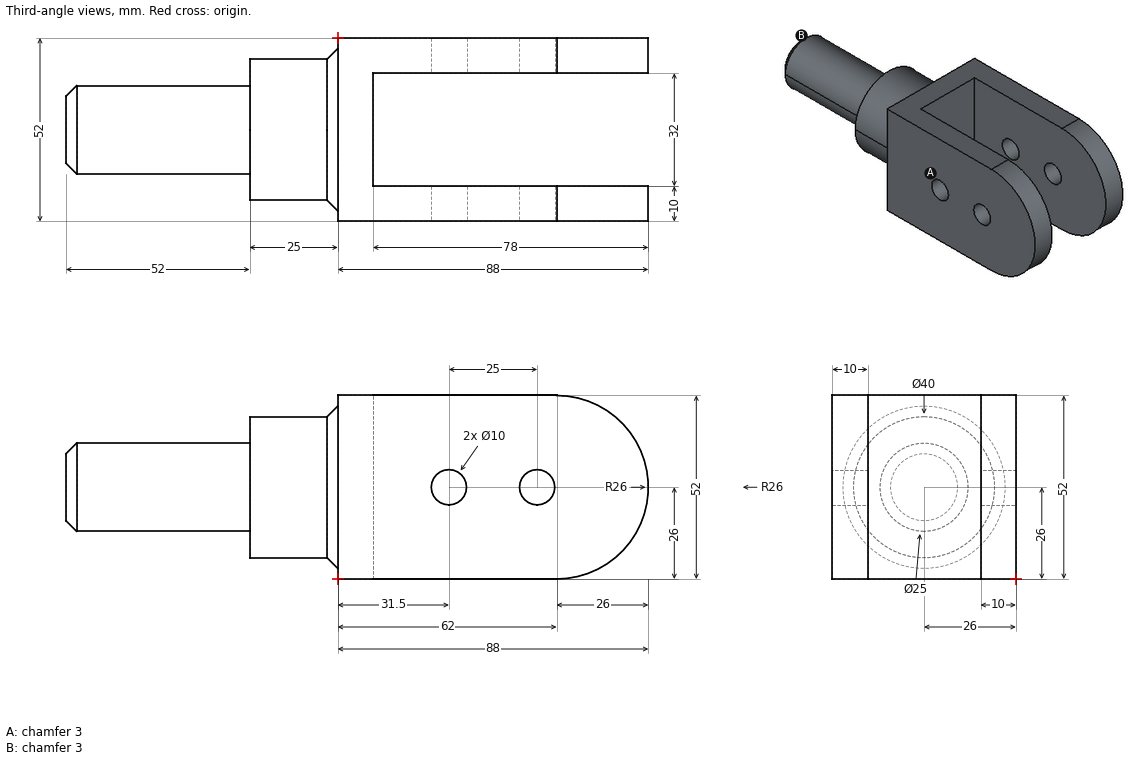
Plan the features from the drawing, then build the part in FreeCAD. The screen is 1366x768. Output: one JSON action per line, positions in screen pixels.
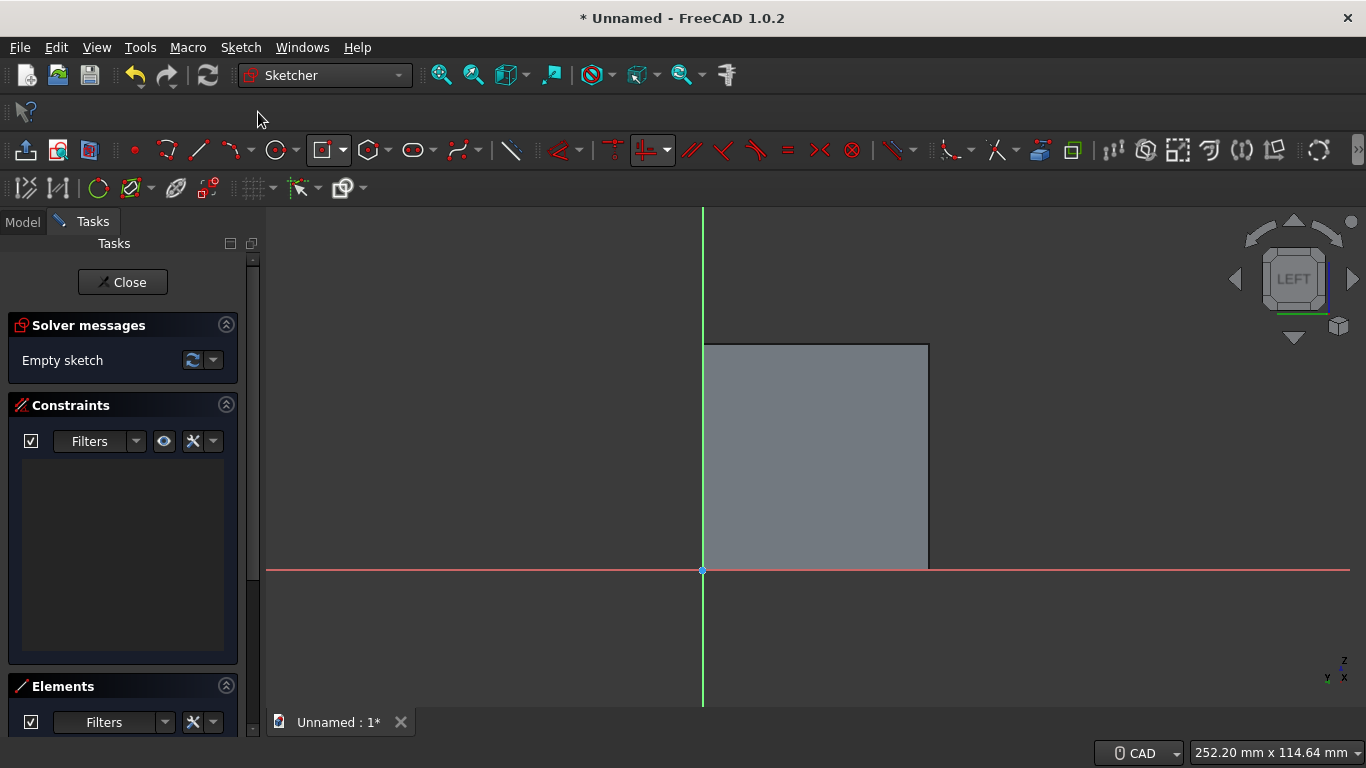
{"action": "scroll", "coordinate": [916, 497], "scroll_direction": "up", "scroll_amount": 2}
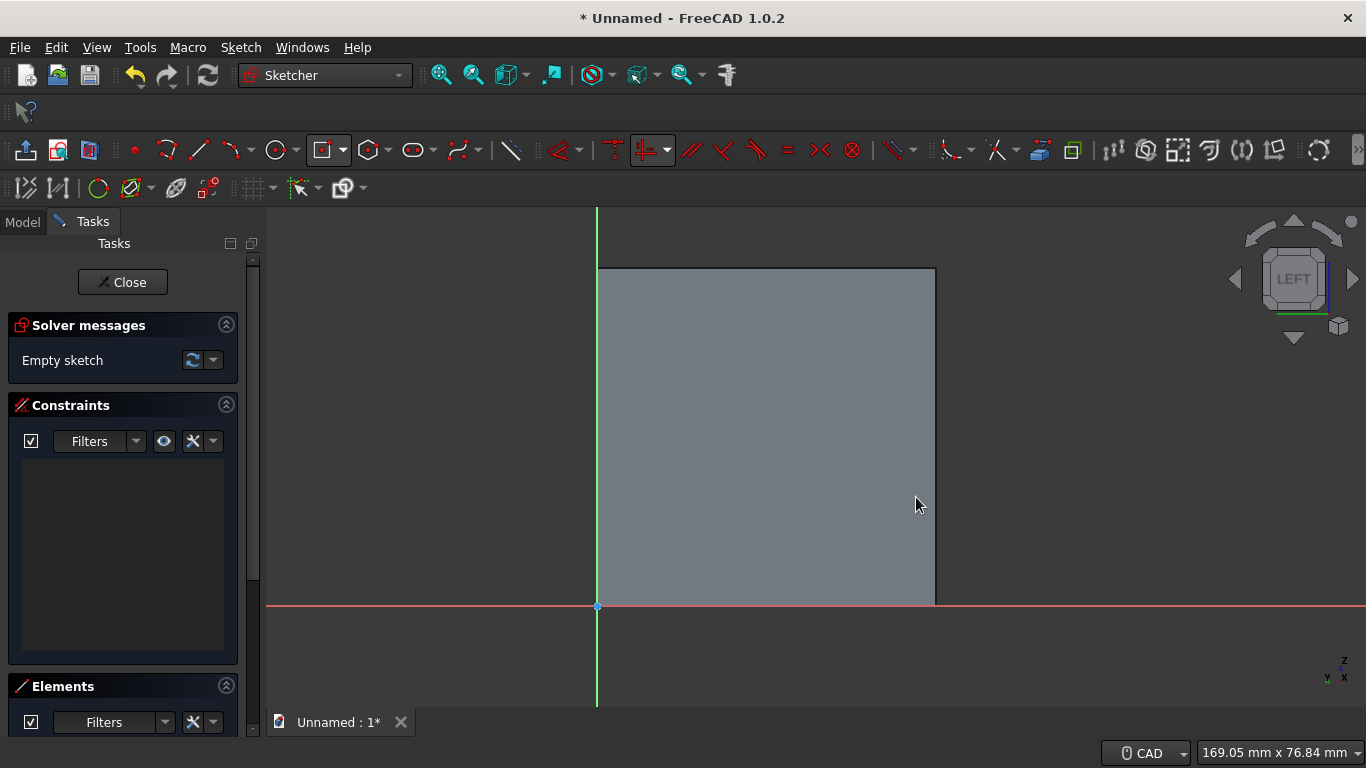
{"action": "left_click", "coordinate": [276, 150]}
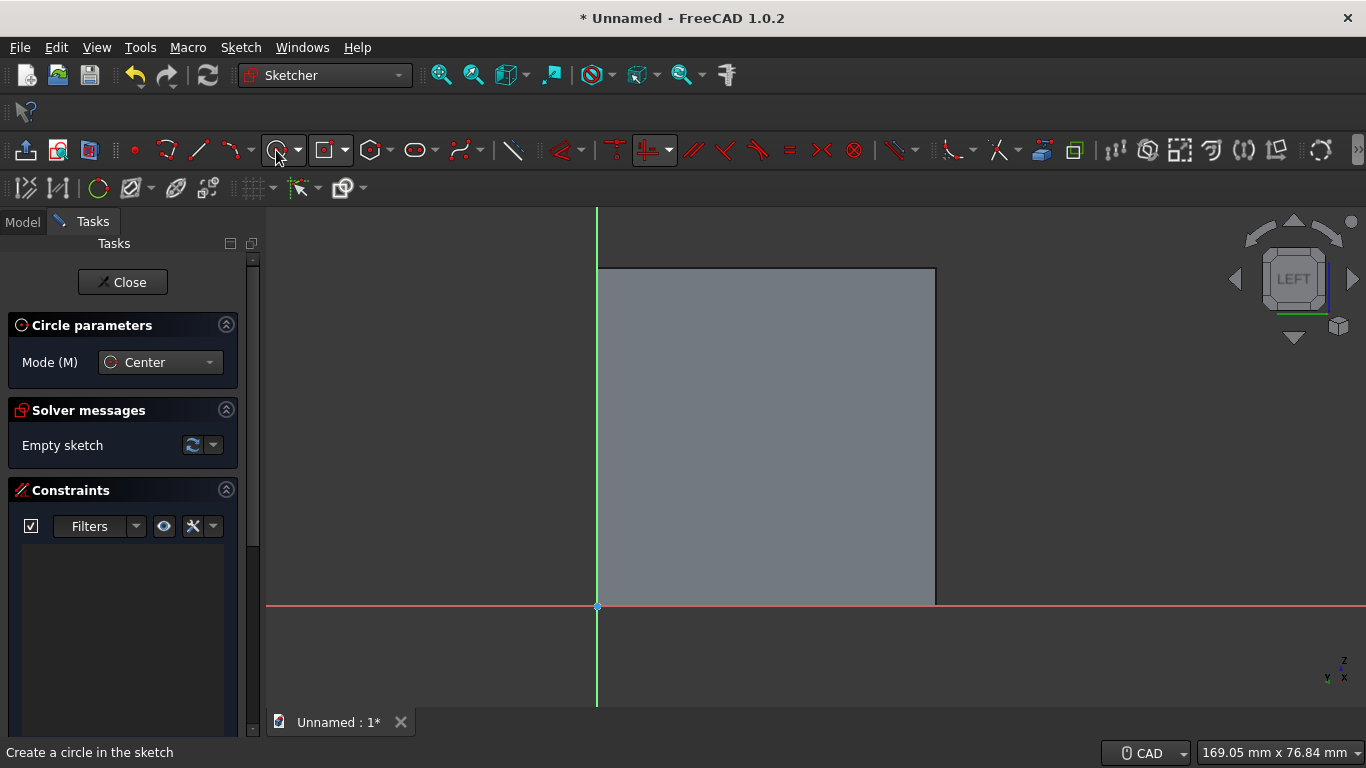
{"action": "left_click", "coordinate": [767, 437]}
{"action": "left_click", "coordinate": [859, 345]}
{"action": "key", "text": "Escape"}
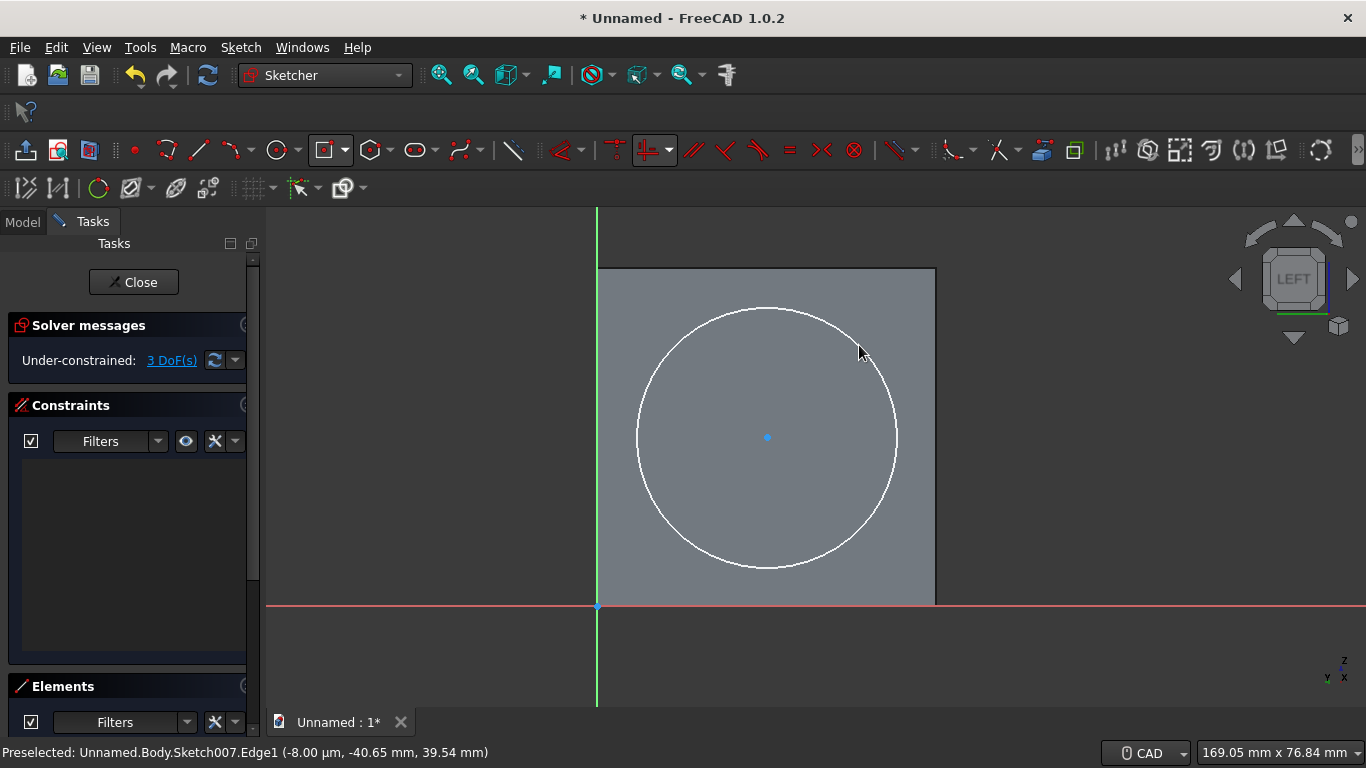
{"action": "left_click", "coordinate": [560, 150]}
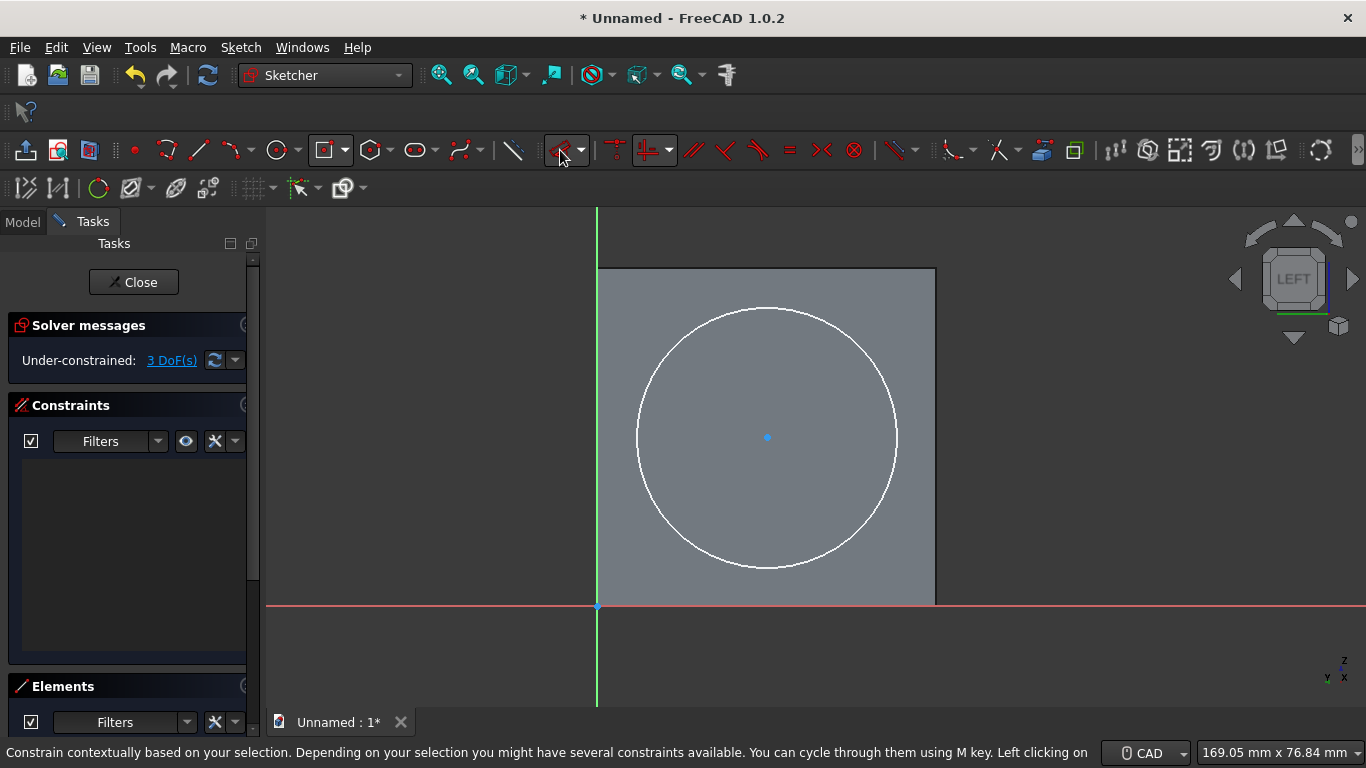
{"action": "left_click", "coordinate": [859, 346]}
{"action": "left_click", "coordinate": [882, 323]}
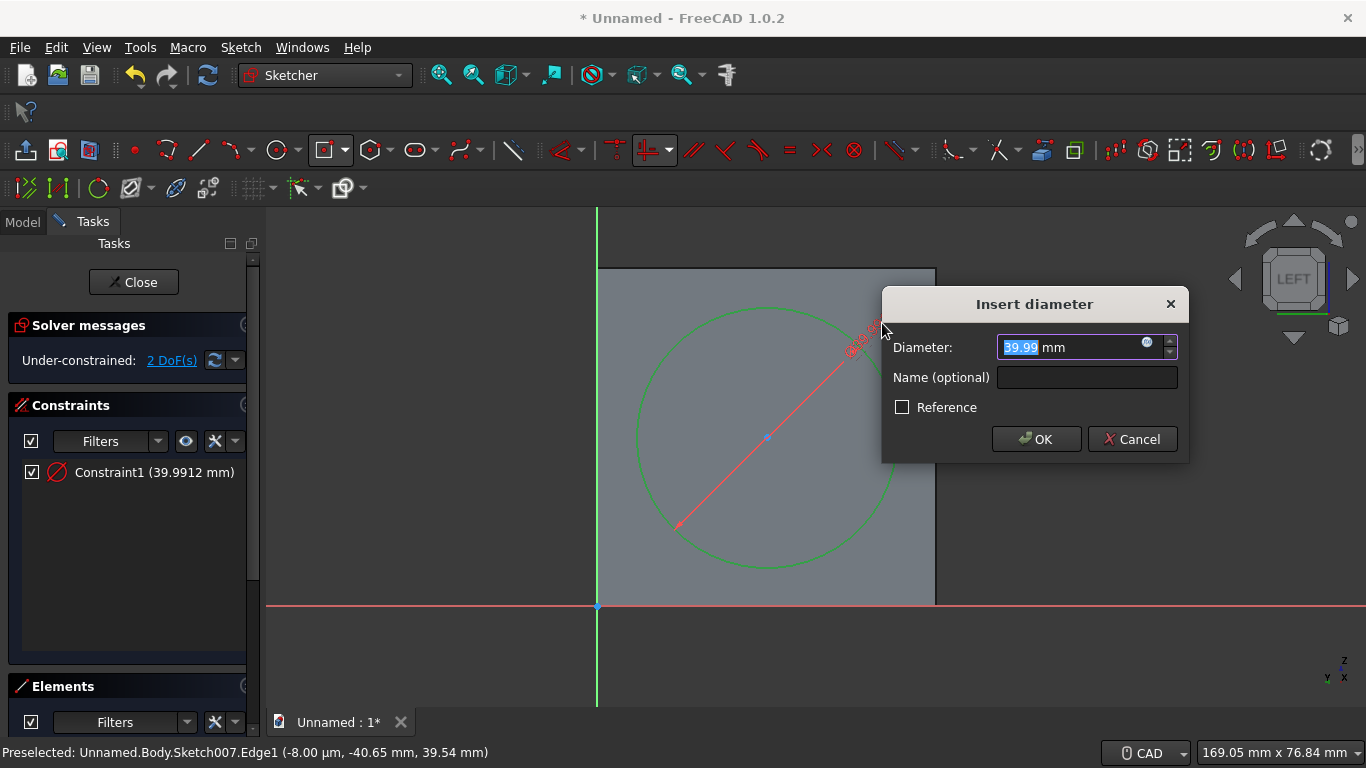
{"action": "type", "text": "40"}
{"action": "key", "text": "Return"}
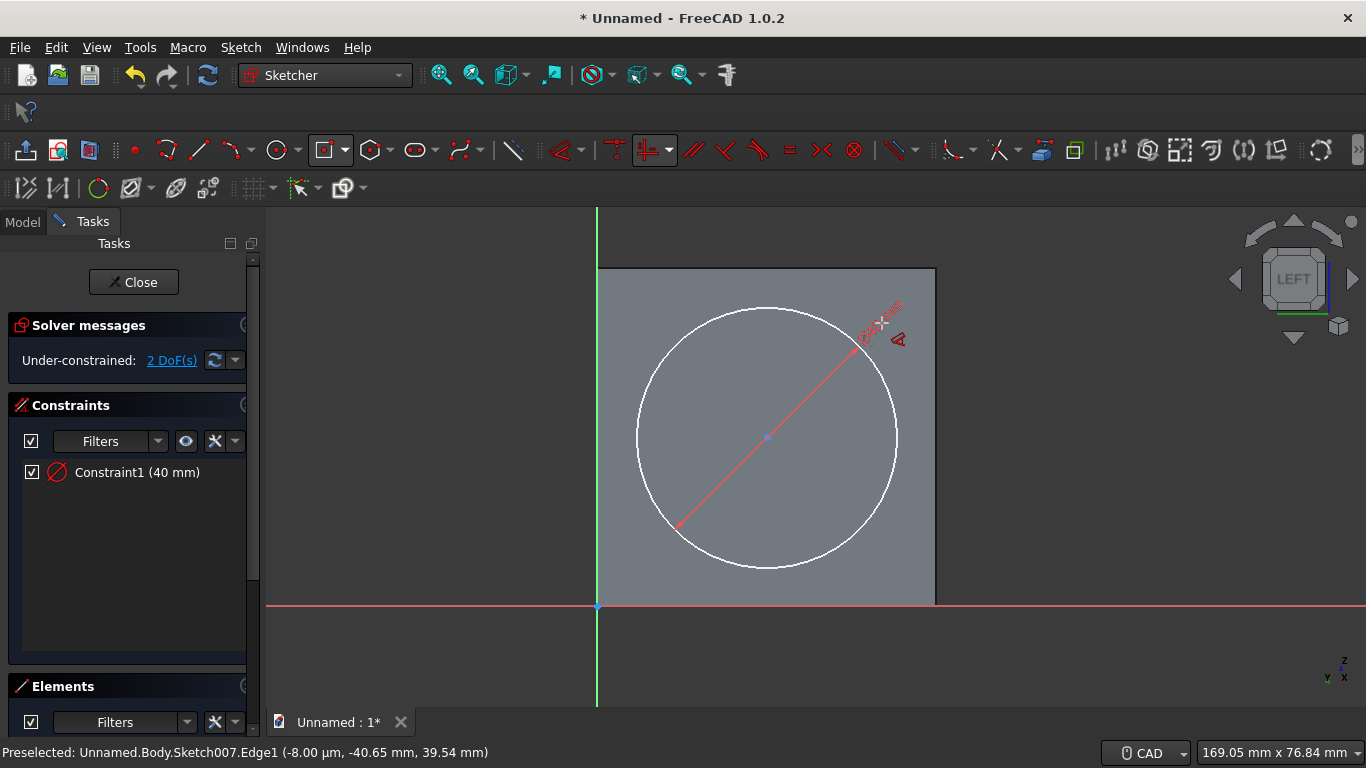
{"action": "left_click", "coordinate": [767, 438]}
{"action": "left_click", "coordinate": [682, 640]}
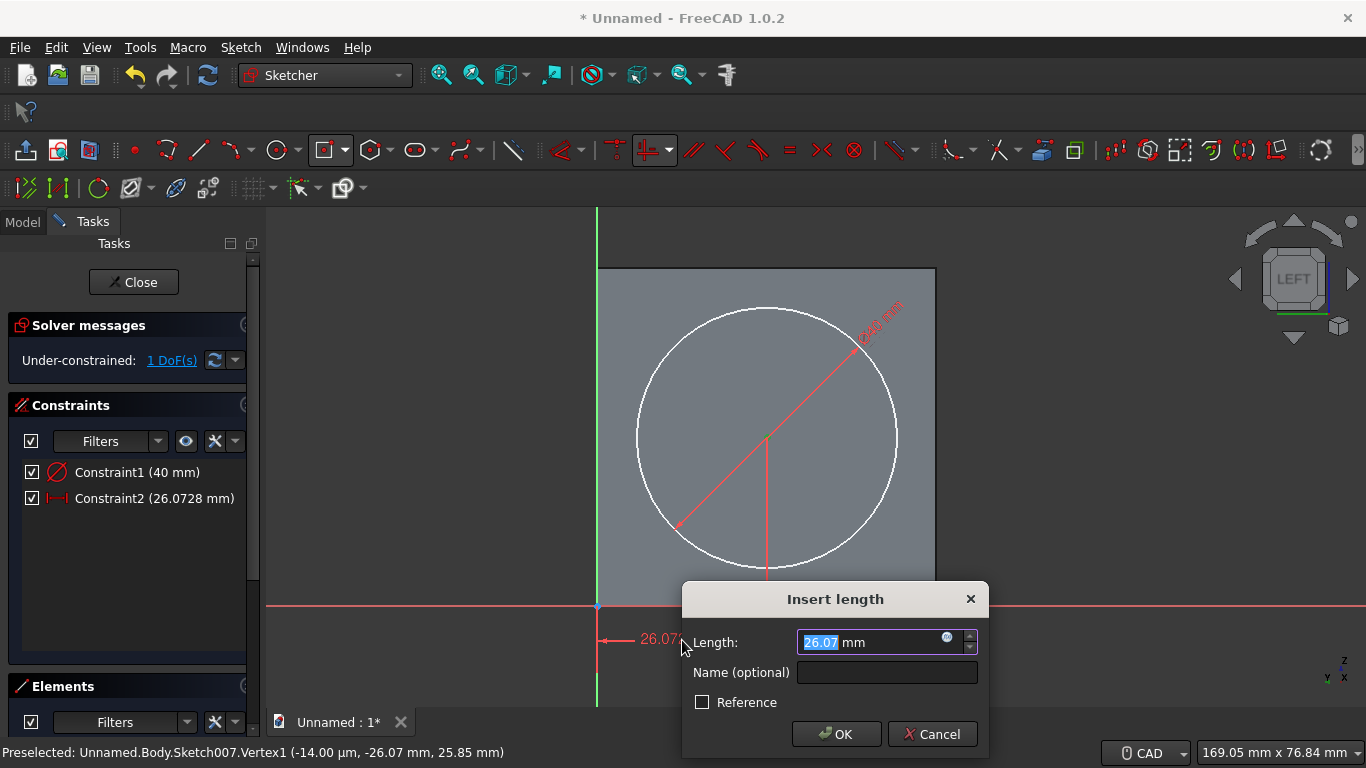
{"action": "type", "text": "26"}
{"action": "key", "text": "Return"}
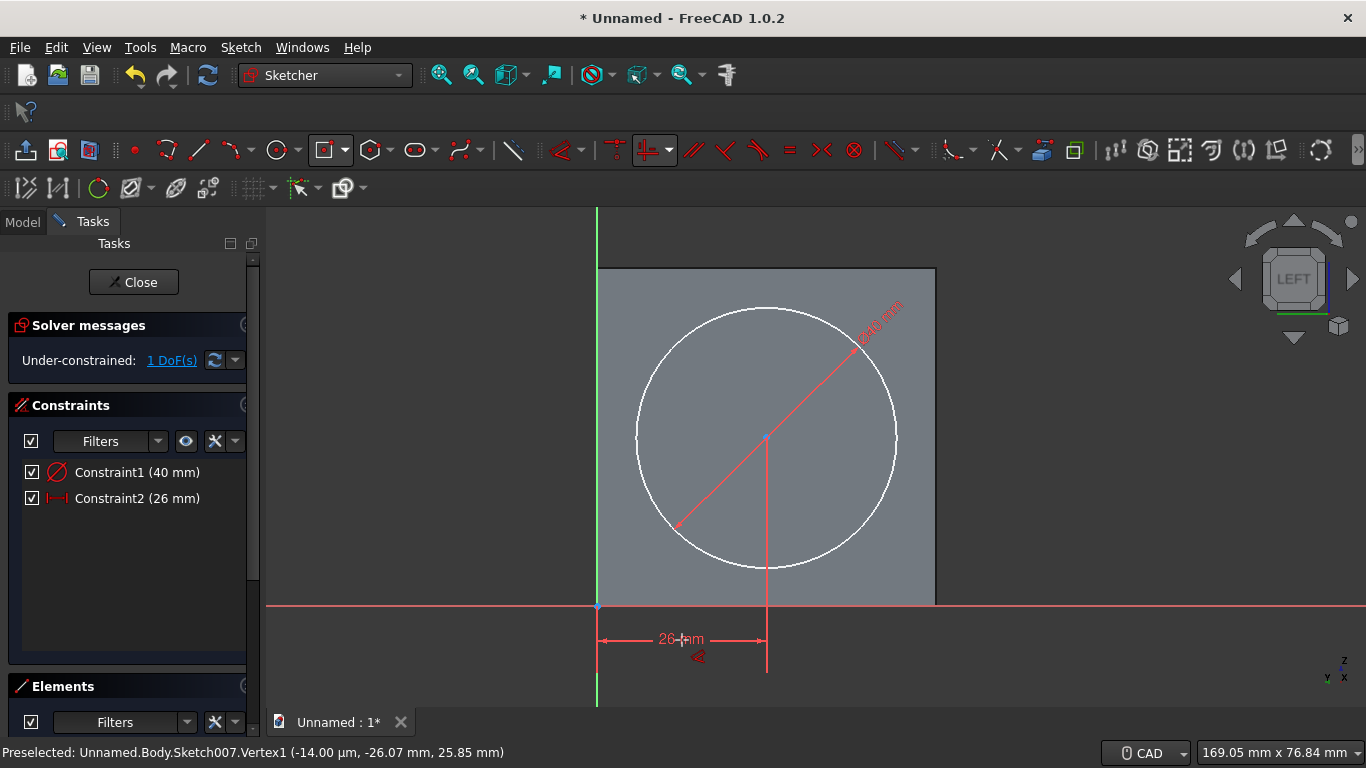
{"action": "left_click", "coordinate": [767, 438]}
{"action": "left_click", "coordinate": [563, 522]}